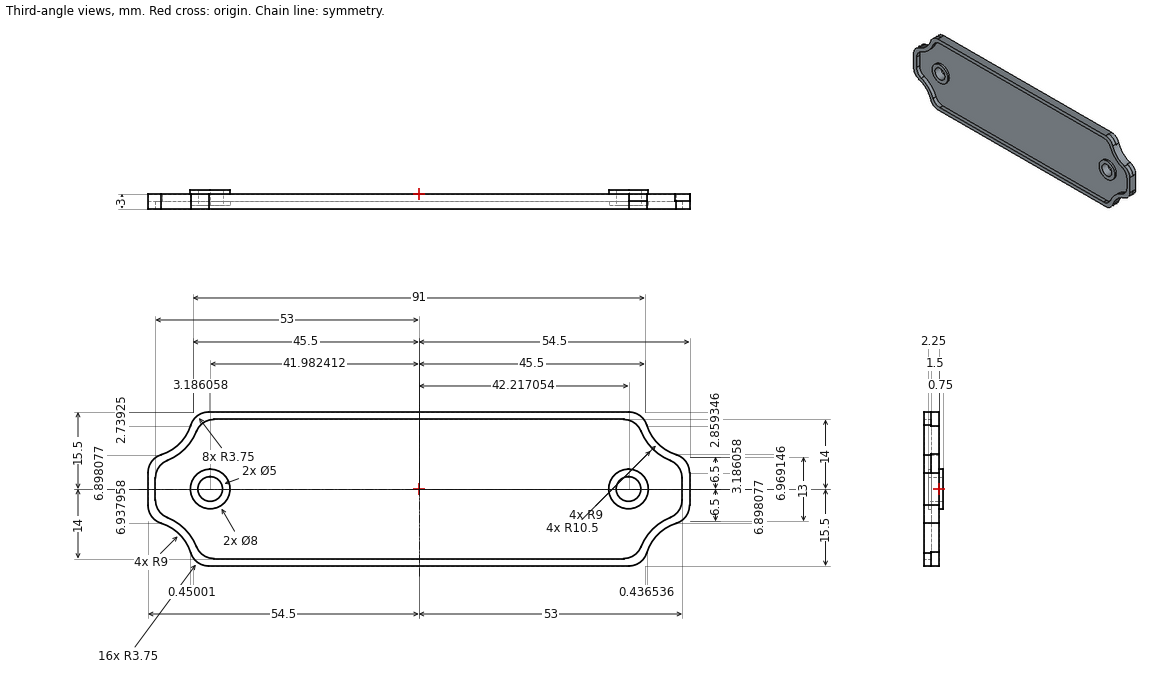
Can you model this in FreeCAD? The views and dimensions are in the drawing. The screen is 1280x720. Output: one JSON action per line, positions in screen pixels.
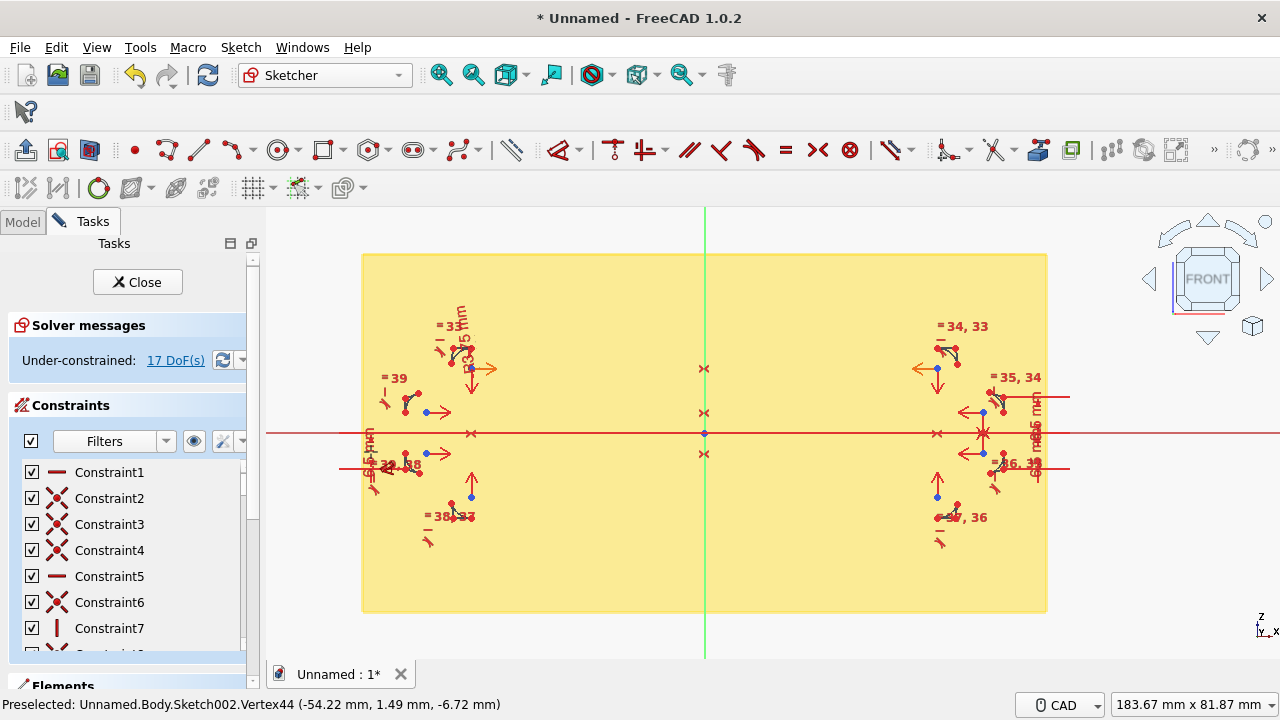
{"action": "left_click", "coordinate": [405, 399]}
{"action": "left_click", "coordinate": [371, 416]}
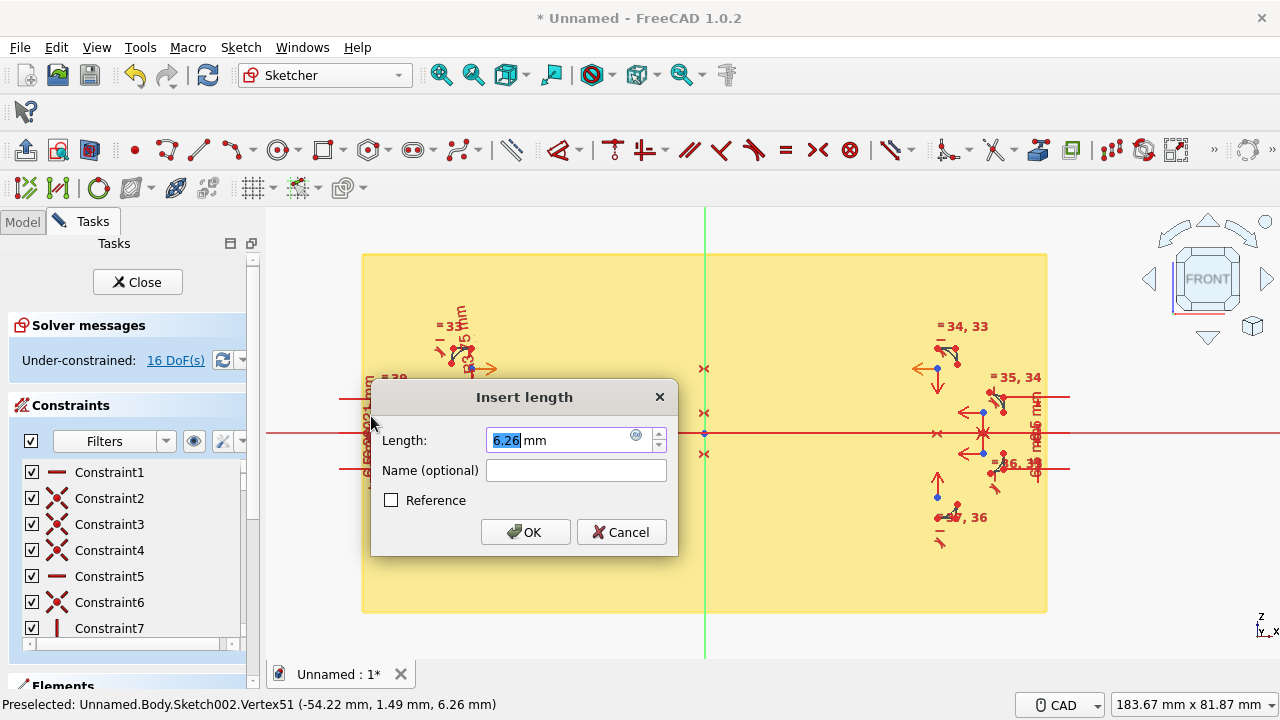
{"action": "type", "text": "6.5"}
{"action": "key", "text": "Return"}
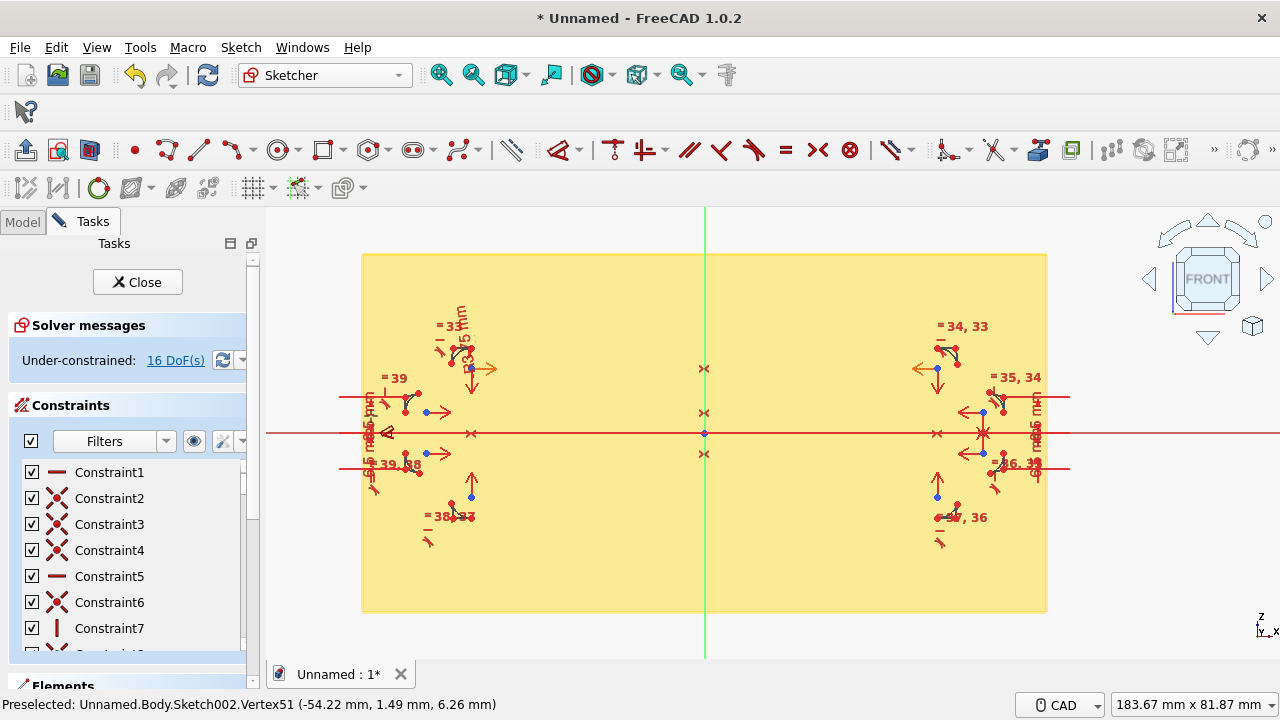
{"action": "left_click", "coordinate": [472, 348]}
{"action": "left_click", "coordinate": [438, 391]}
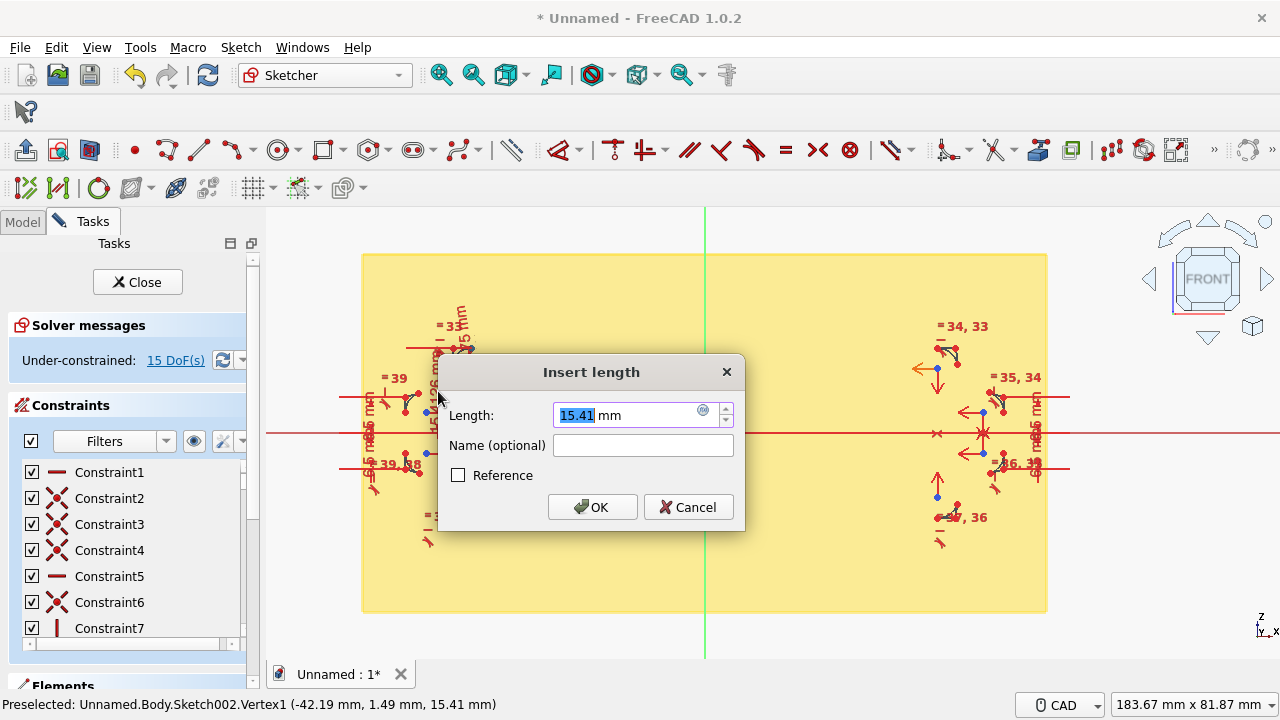
{"action": "type", "text": "15.5"}
{"action": "key", "text": "Return"}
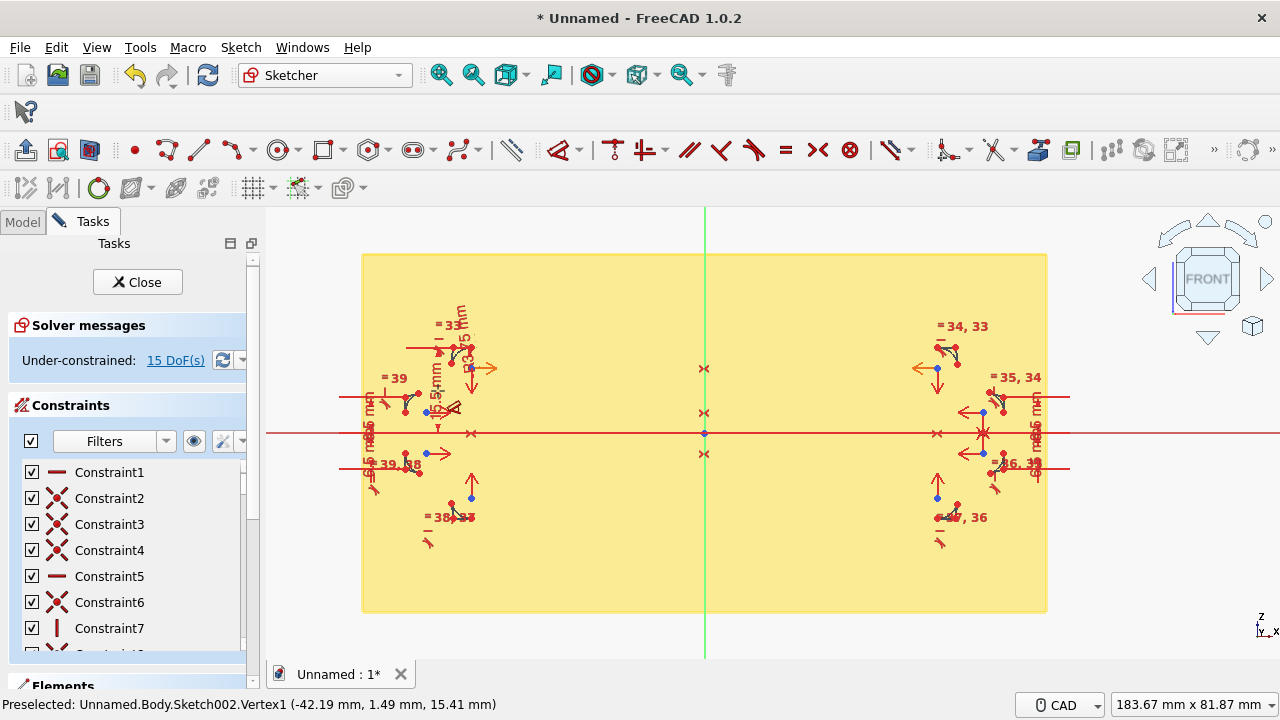
{"action": "left_click", "coordinate": [453, 348]}
{"action": "left_click", "coordinate": [579, 314]}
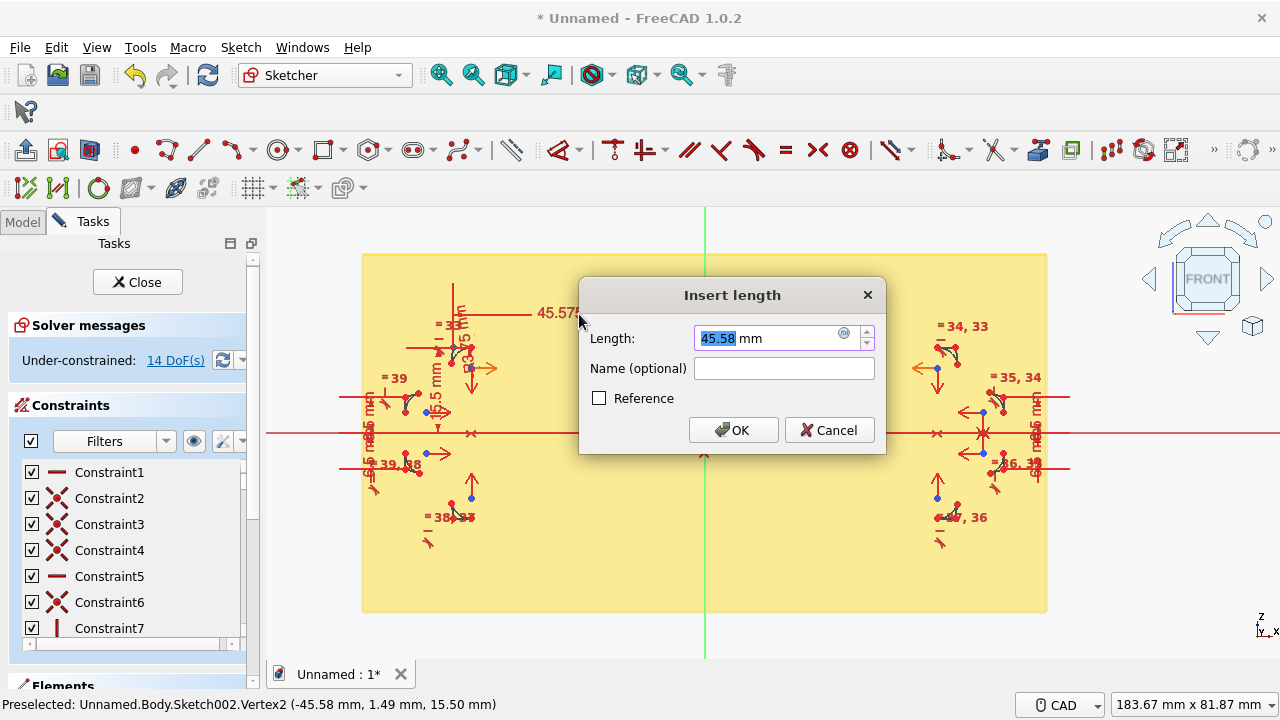
{"action": "type", "text": "45.5"}
{"action": "key", "text": "Return"}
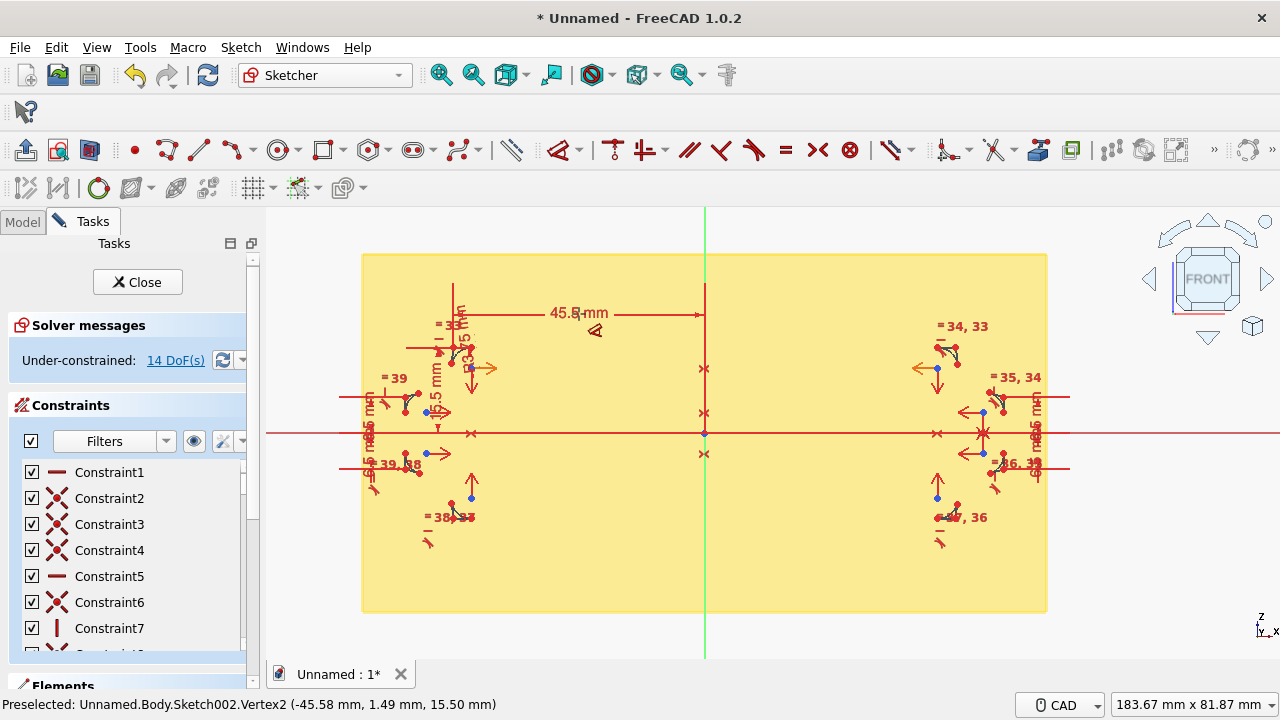
{"action": "left_click", "coordinate": [956, 348]}
{"action": "left_click", "coordinate": [830, 314]}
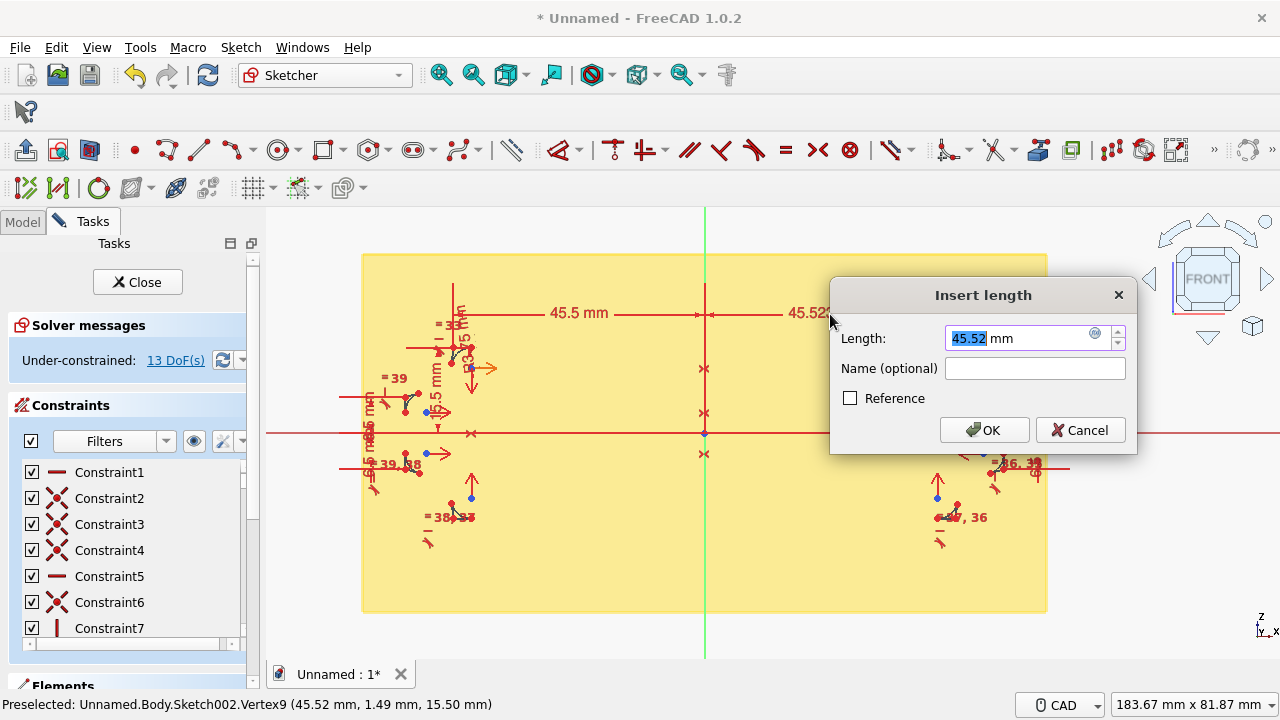
{"action": "type", "text": "45.5"}
{"action": "key", "text": "Return"}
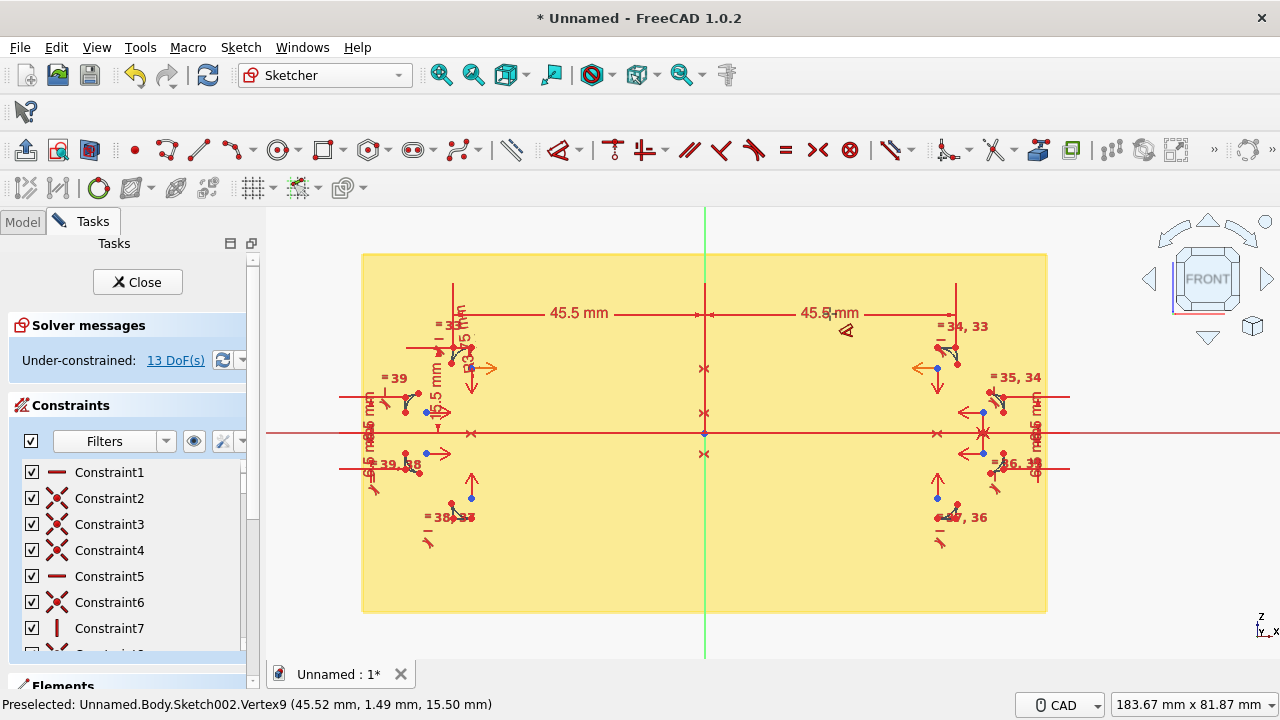
{"action": "left_click", "coordinate": [1004, 413]}
{"action": "left_click", "coordinate": [854, 379]}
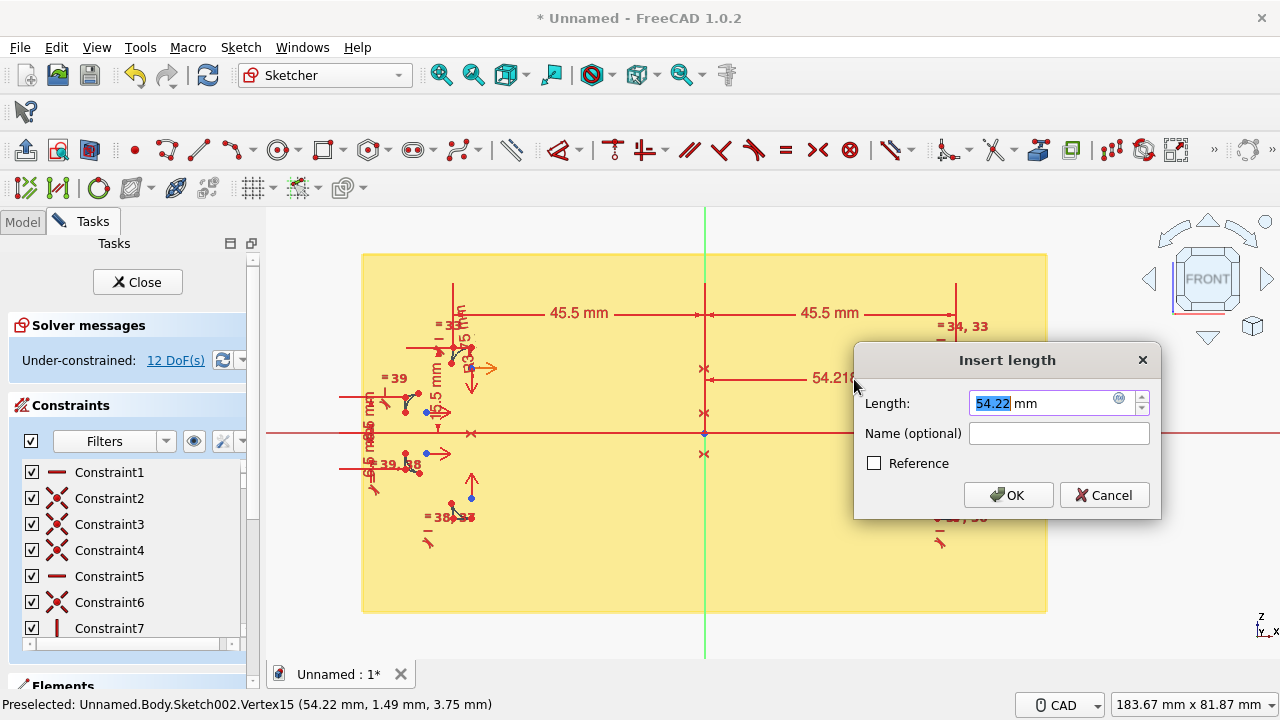
{"action": "type", "text": "54.5"}
{"action": "key", "text": "Return"}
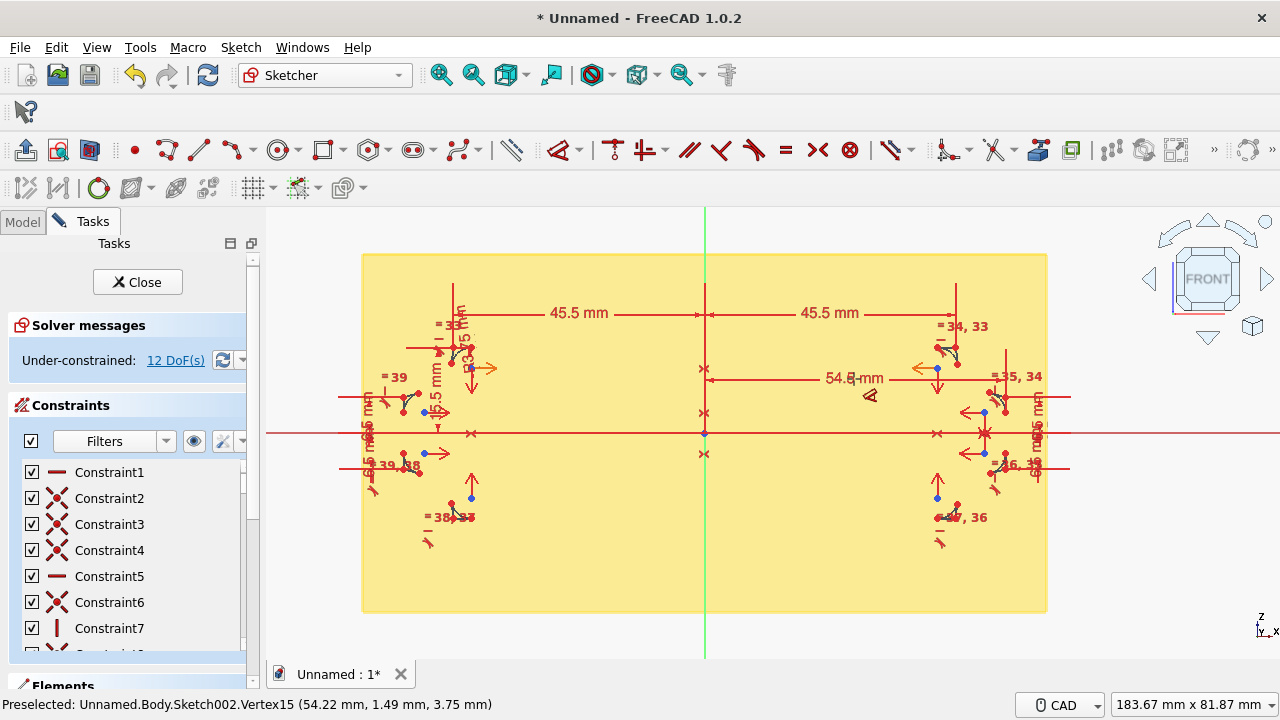
{"action": "left_click", "coordinate": [955, 519]}
{"action": "left_click", "coordinate": [830, 553]}